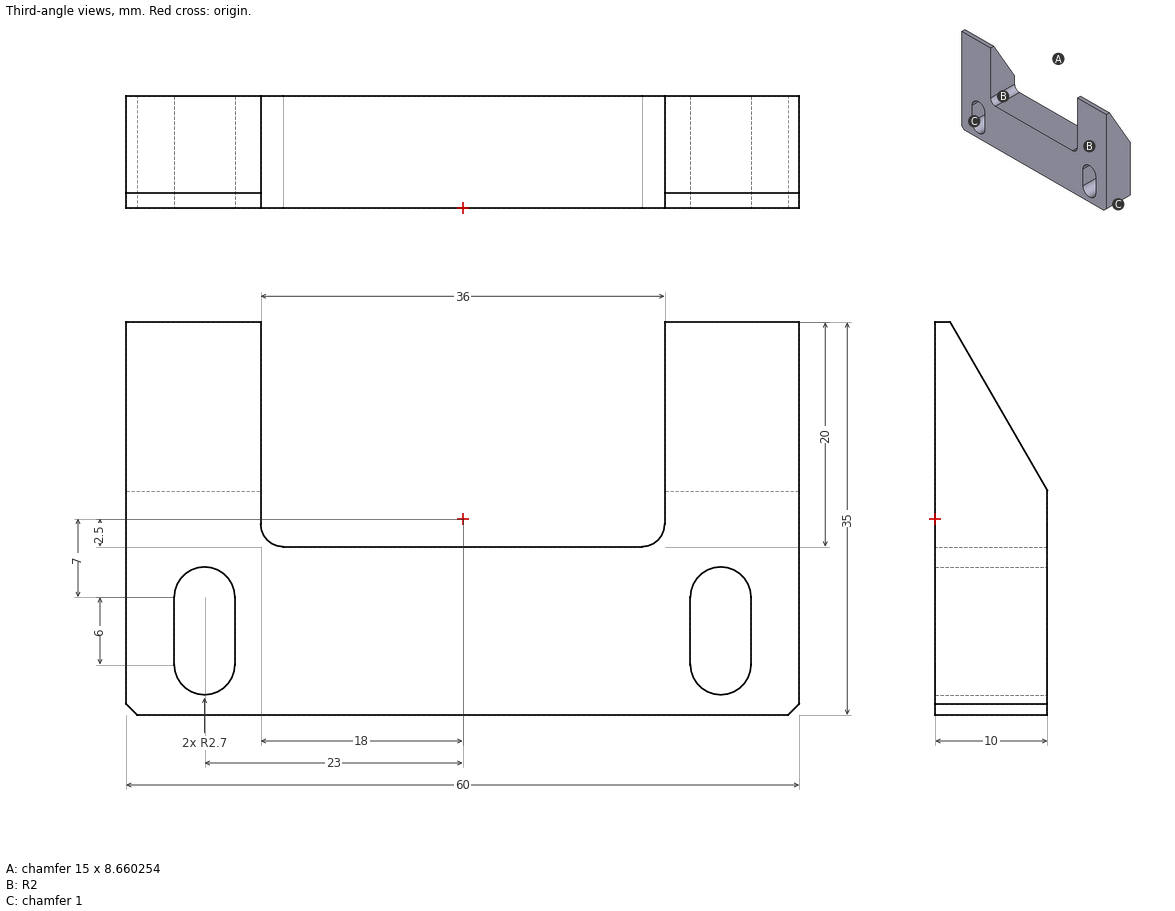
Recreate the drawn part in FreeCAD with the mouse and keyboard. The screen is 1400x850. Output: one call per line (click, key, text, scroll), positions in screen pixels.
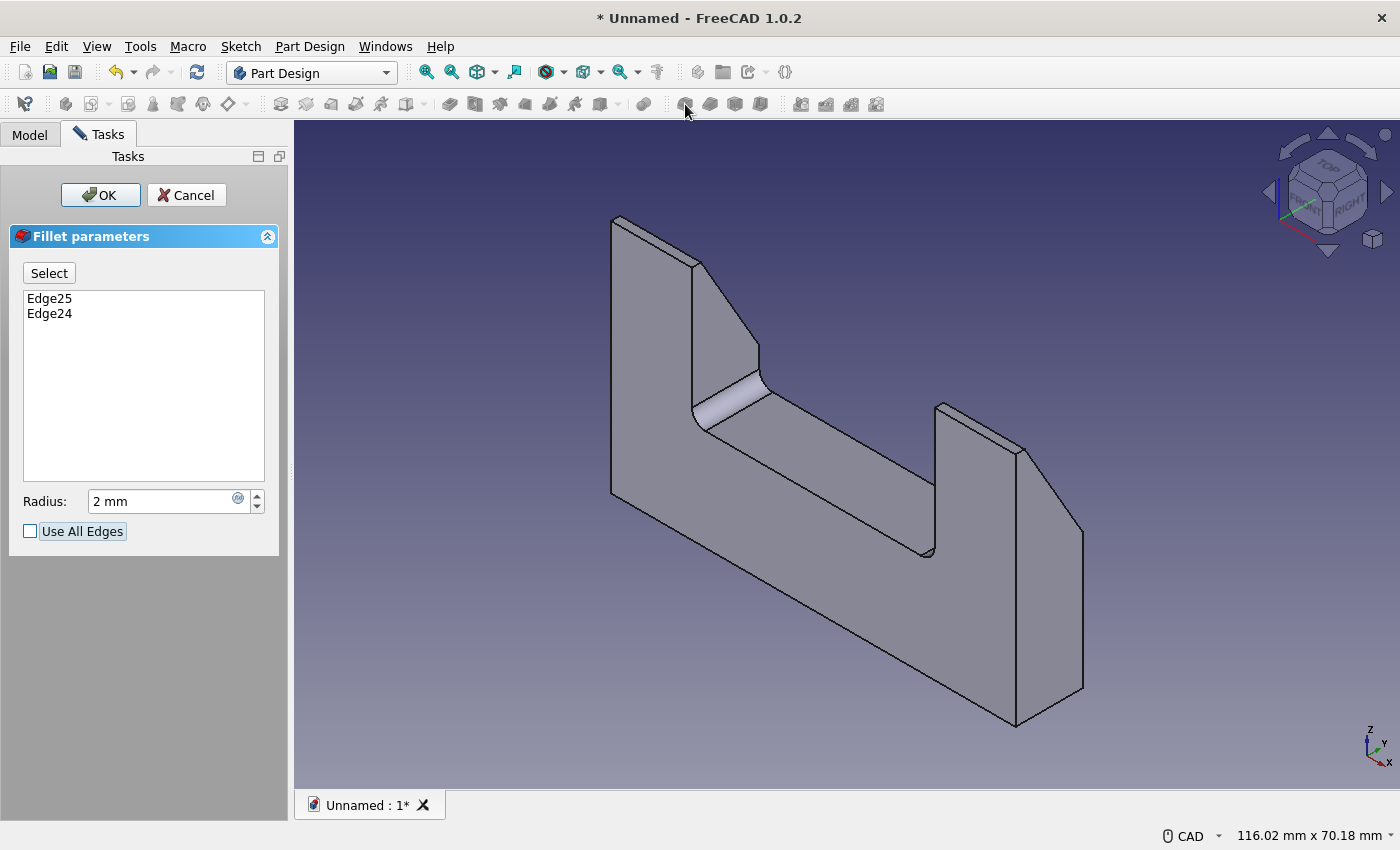
click(101, 195)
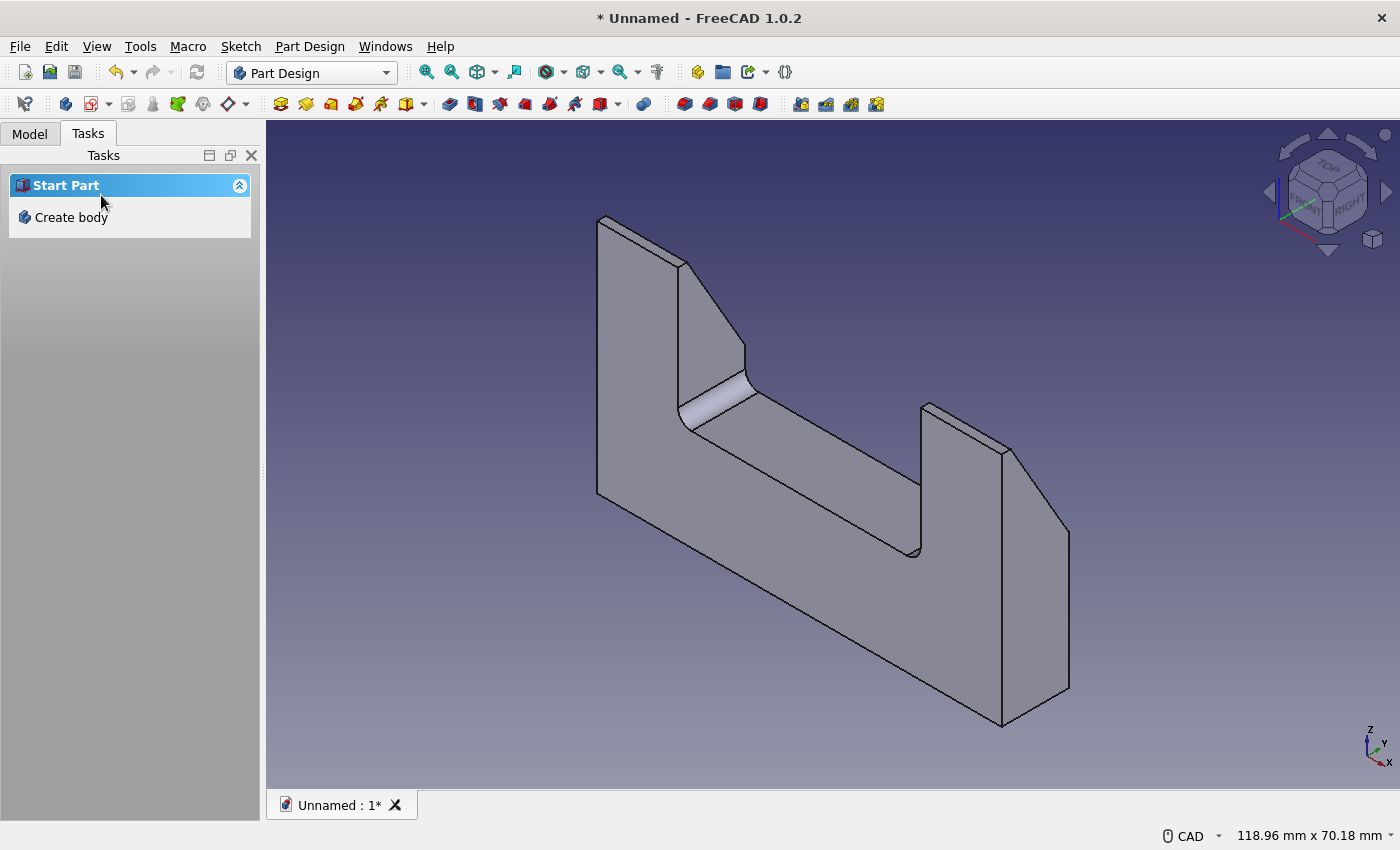
key(4)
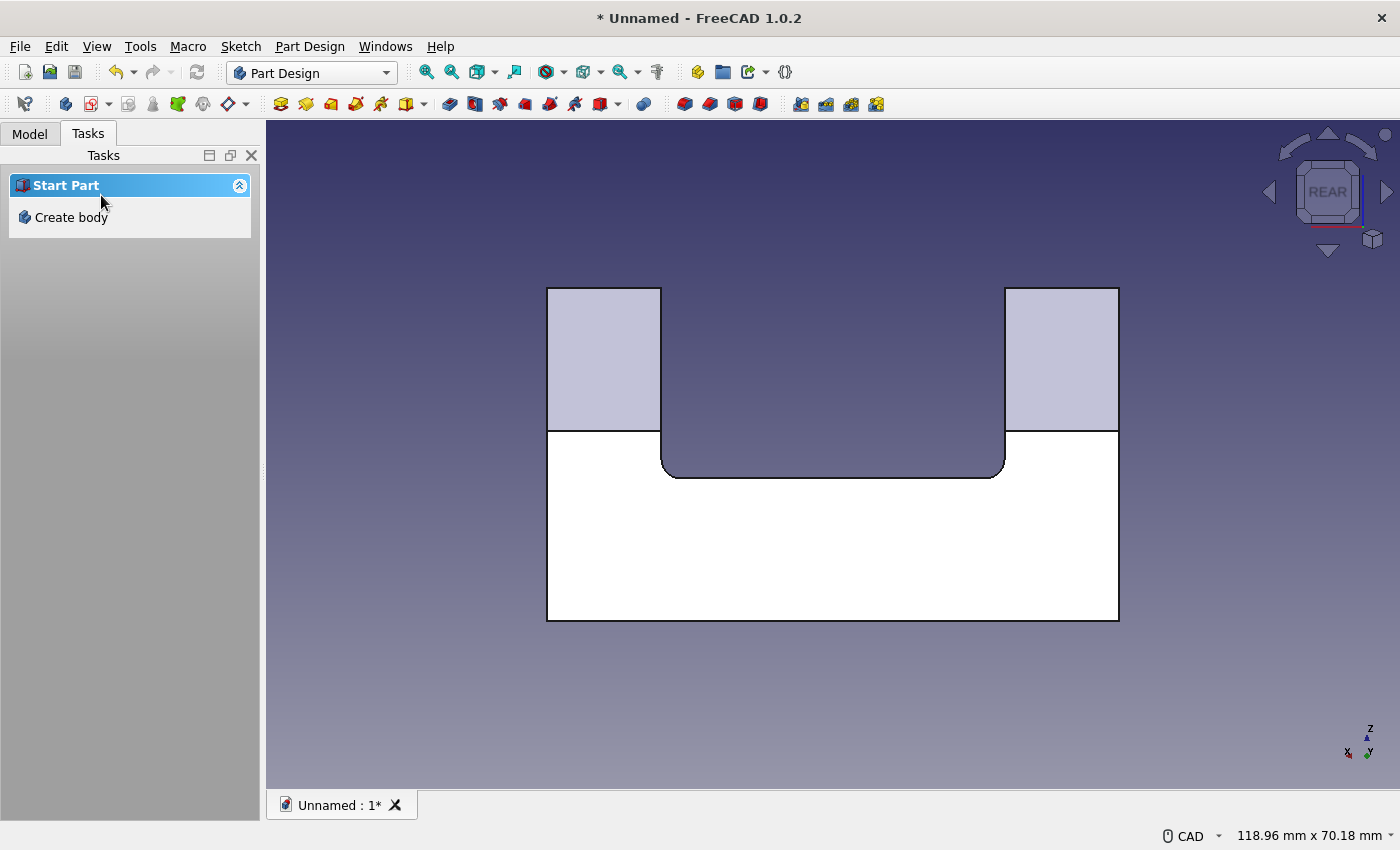
click(670, 552)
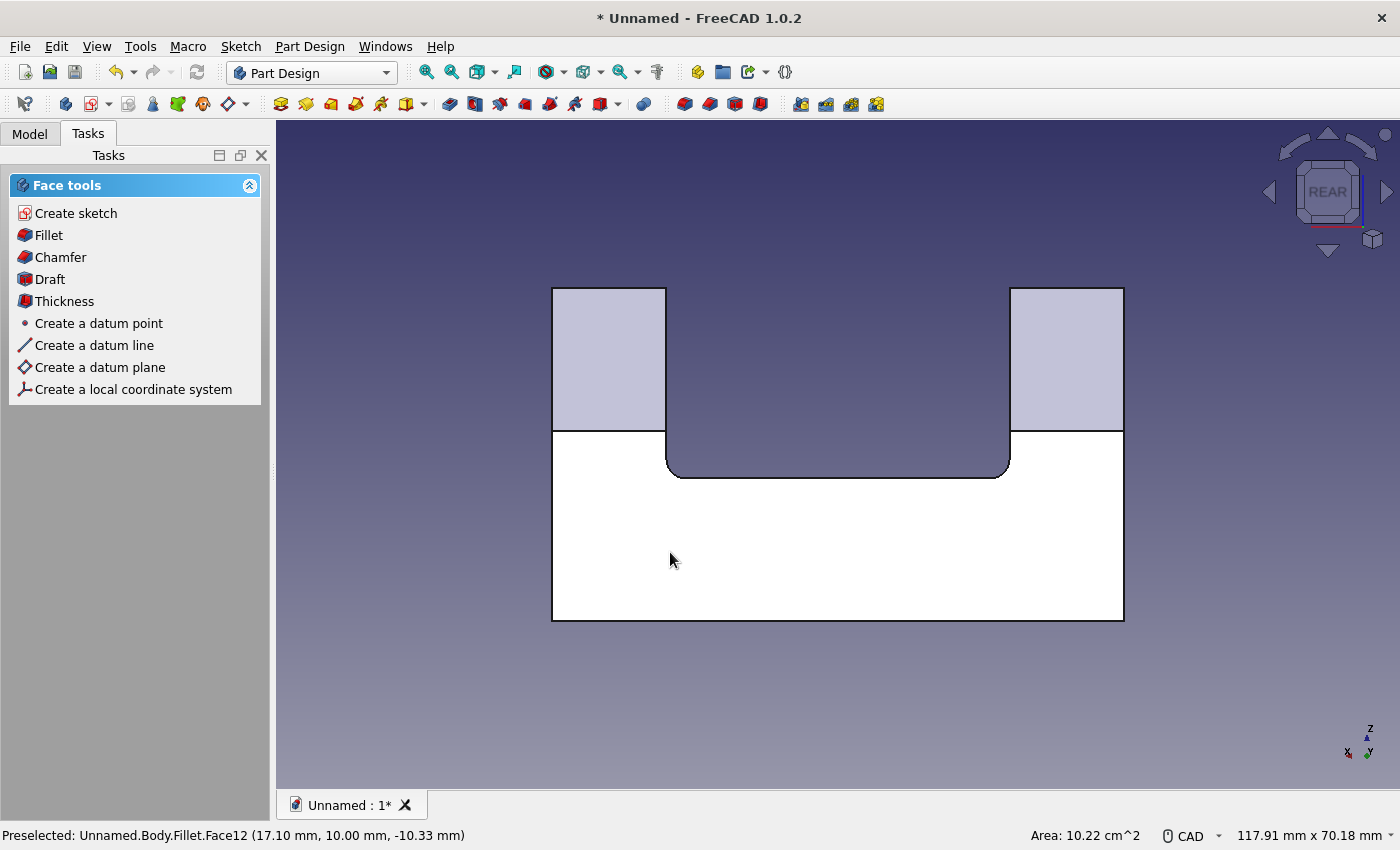
click(90, 104)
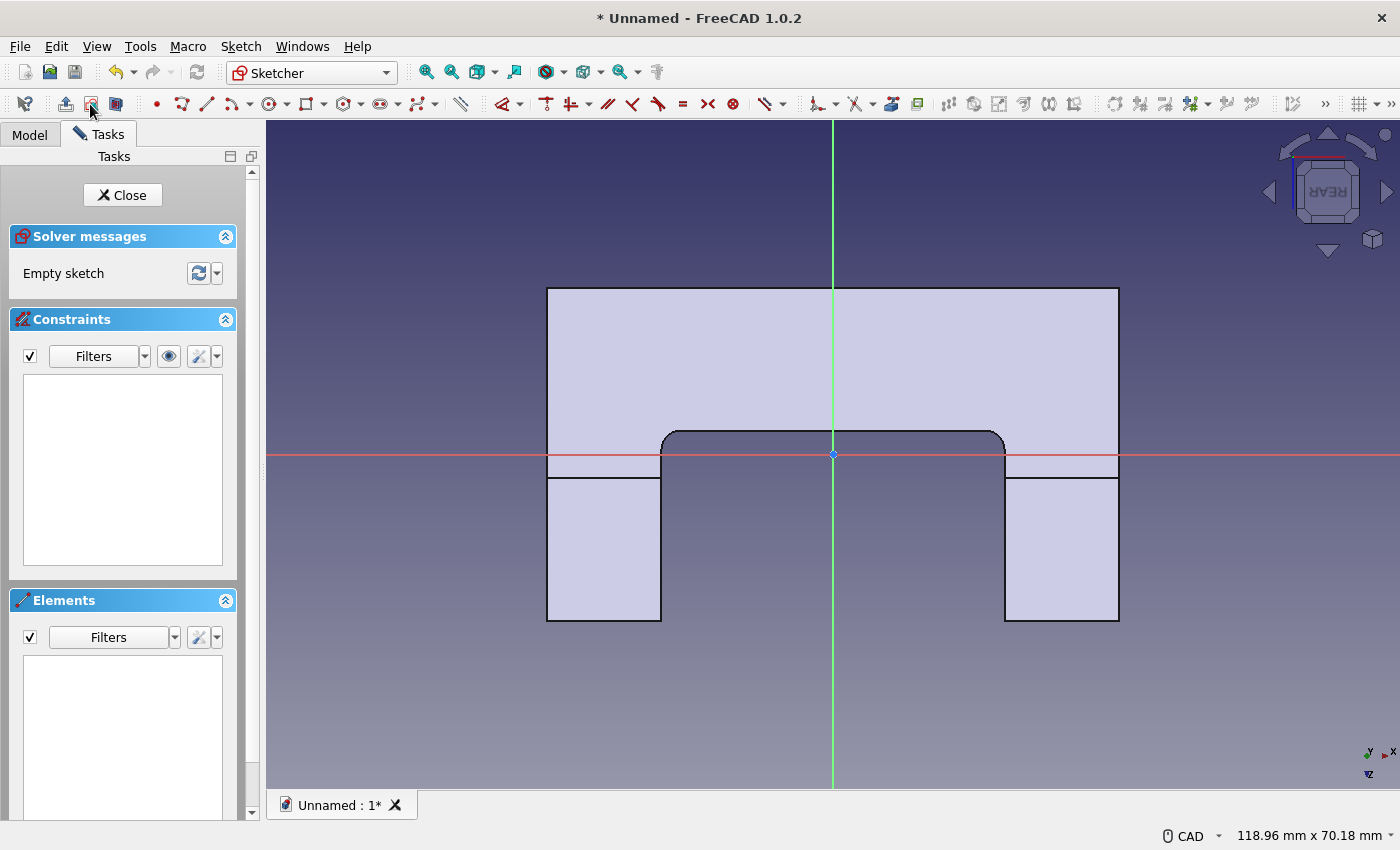
scroll(679, 336, up, 5)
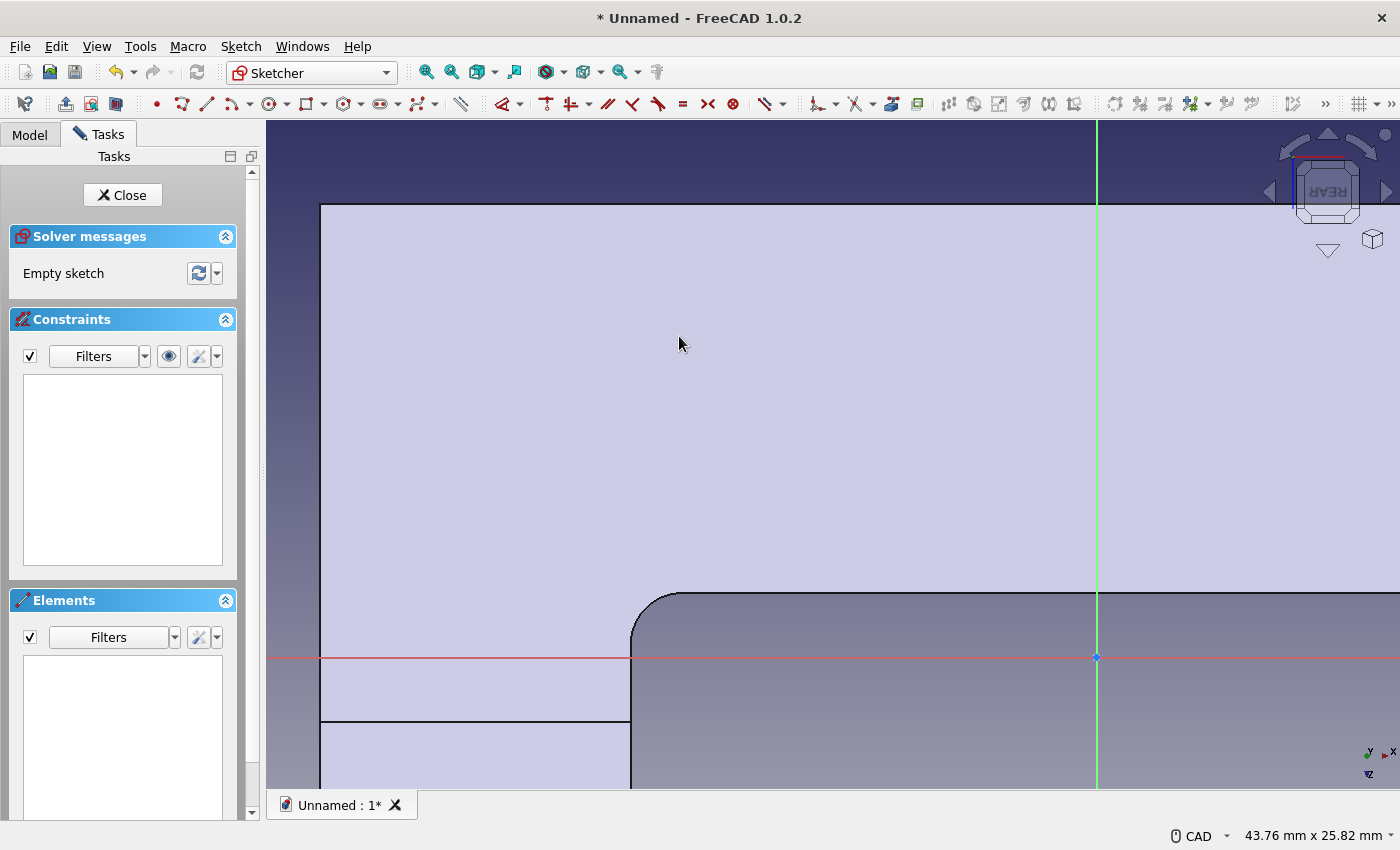
key(g)
key(s)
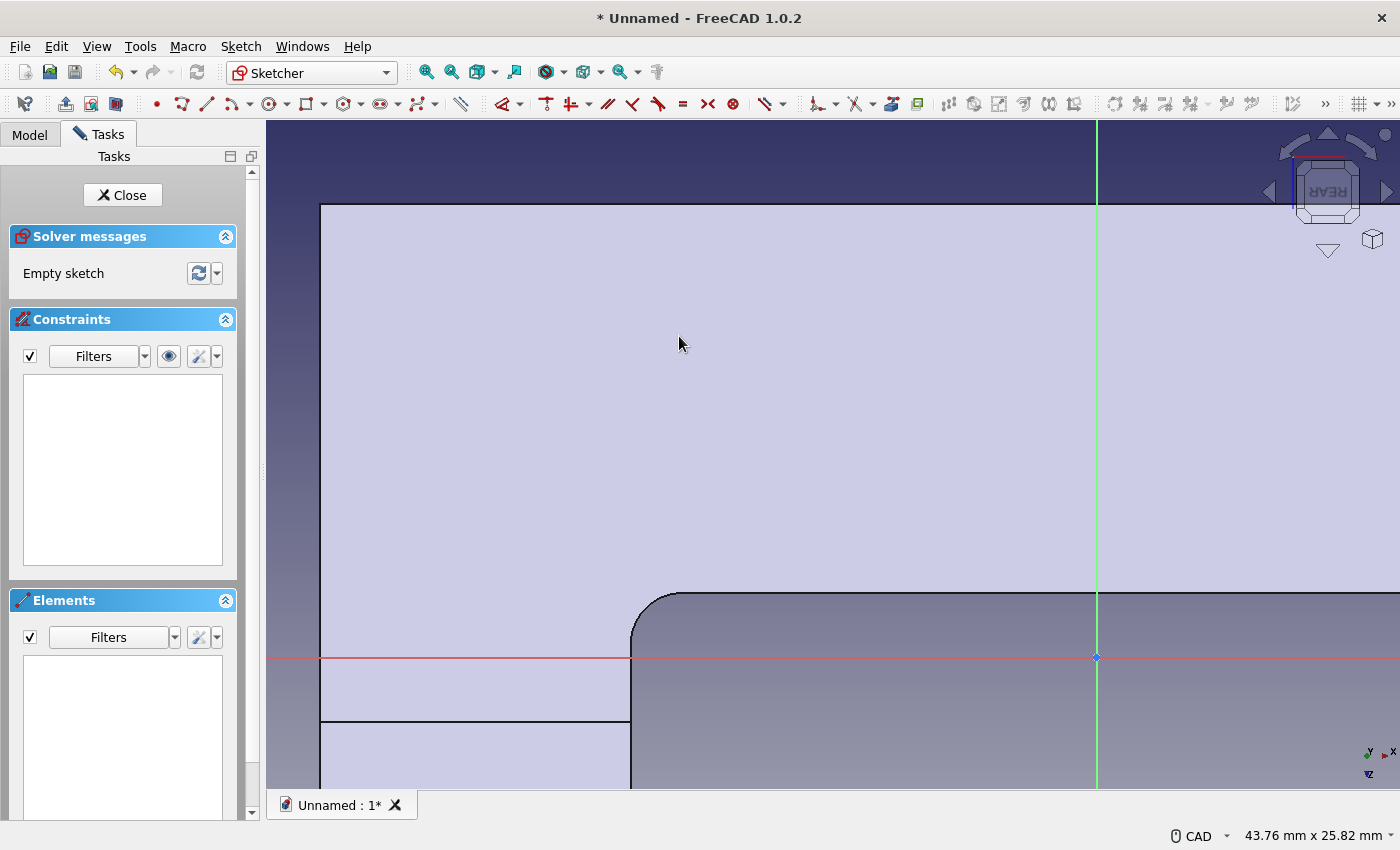
click(501, 476)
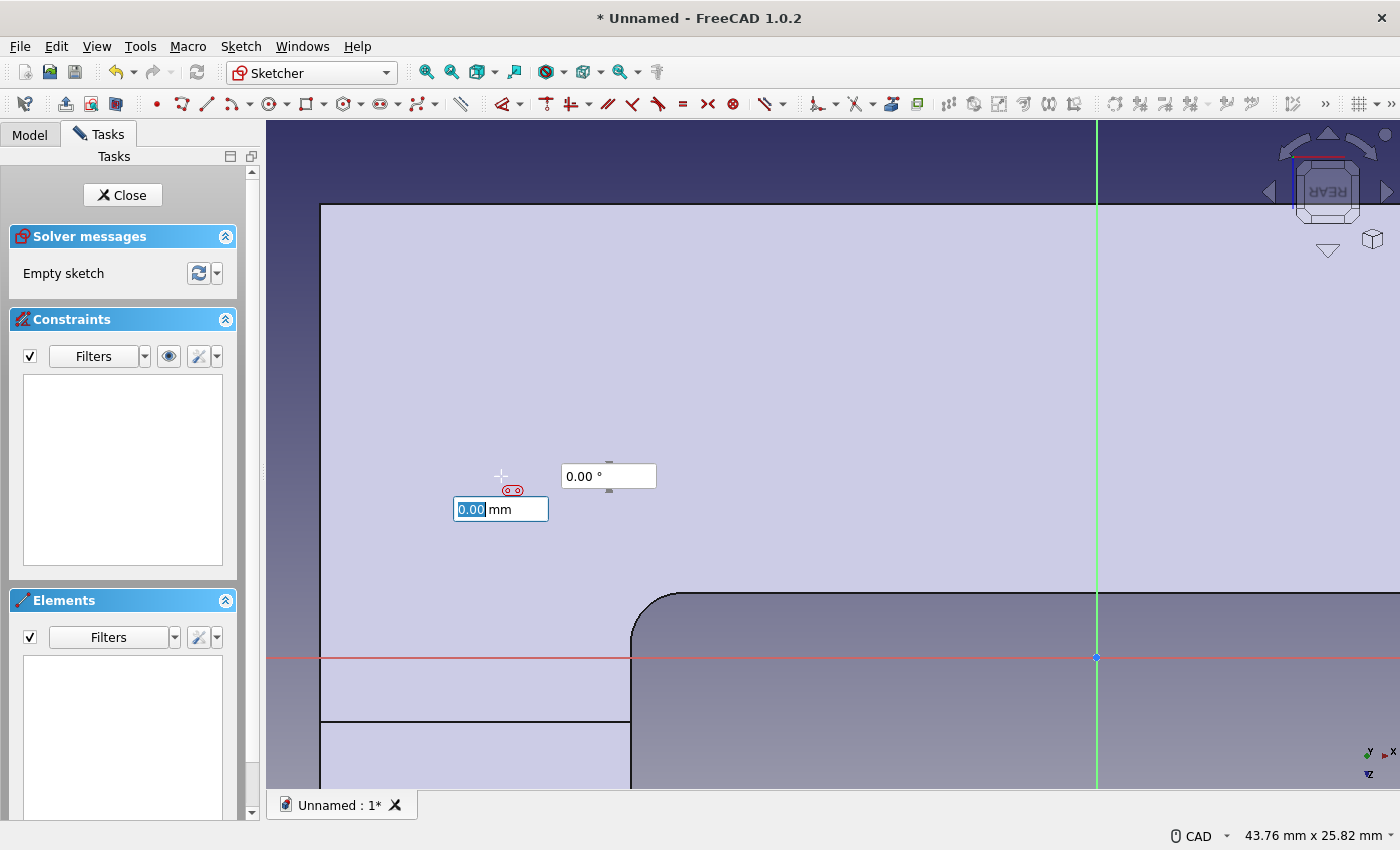
click(501, 321)